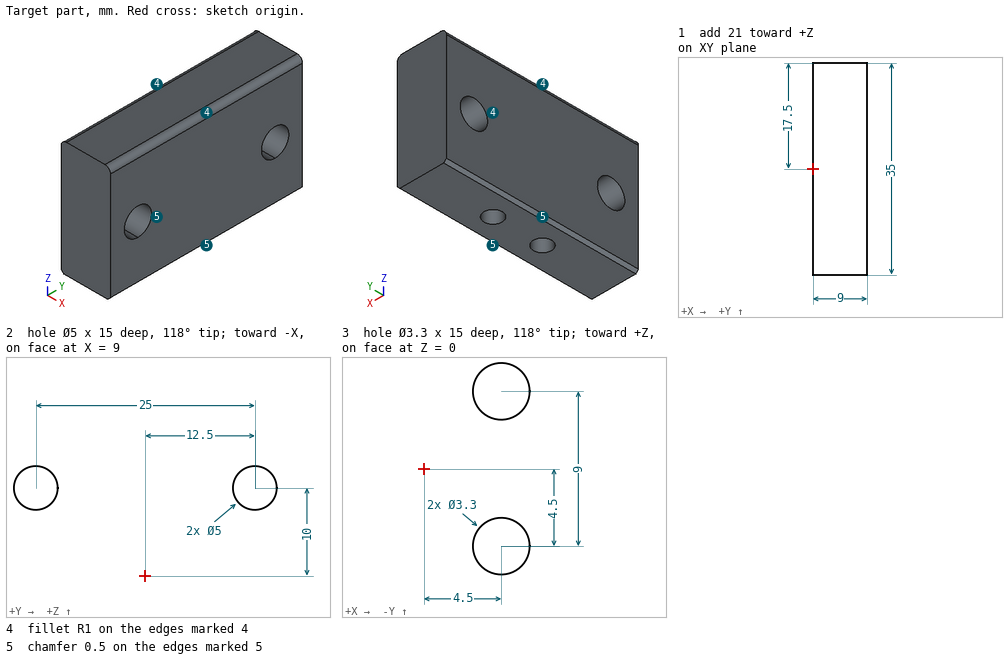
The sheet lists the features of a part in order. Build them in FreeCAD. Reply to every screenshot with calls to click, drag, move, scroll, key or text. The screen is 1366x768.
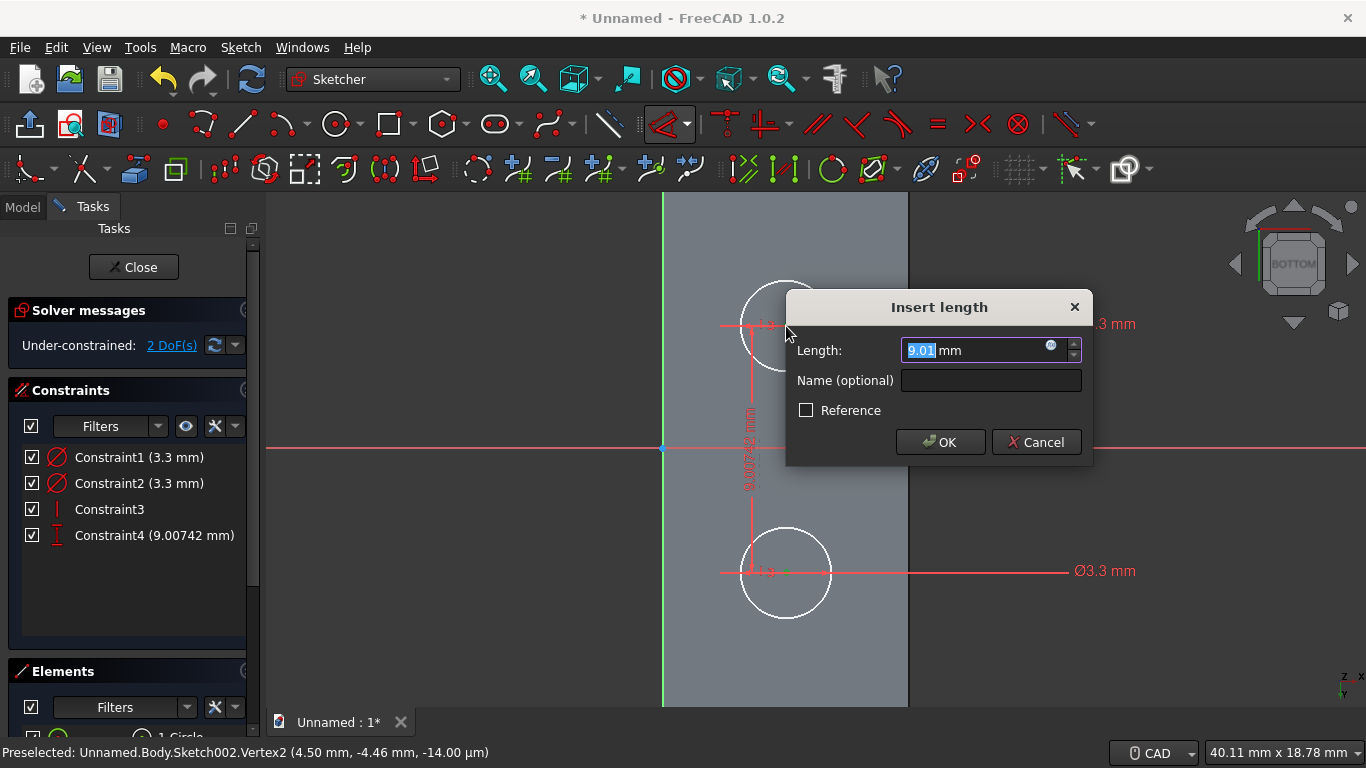
text(9)
key(Return)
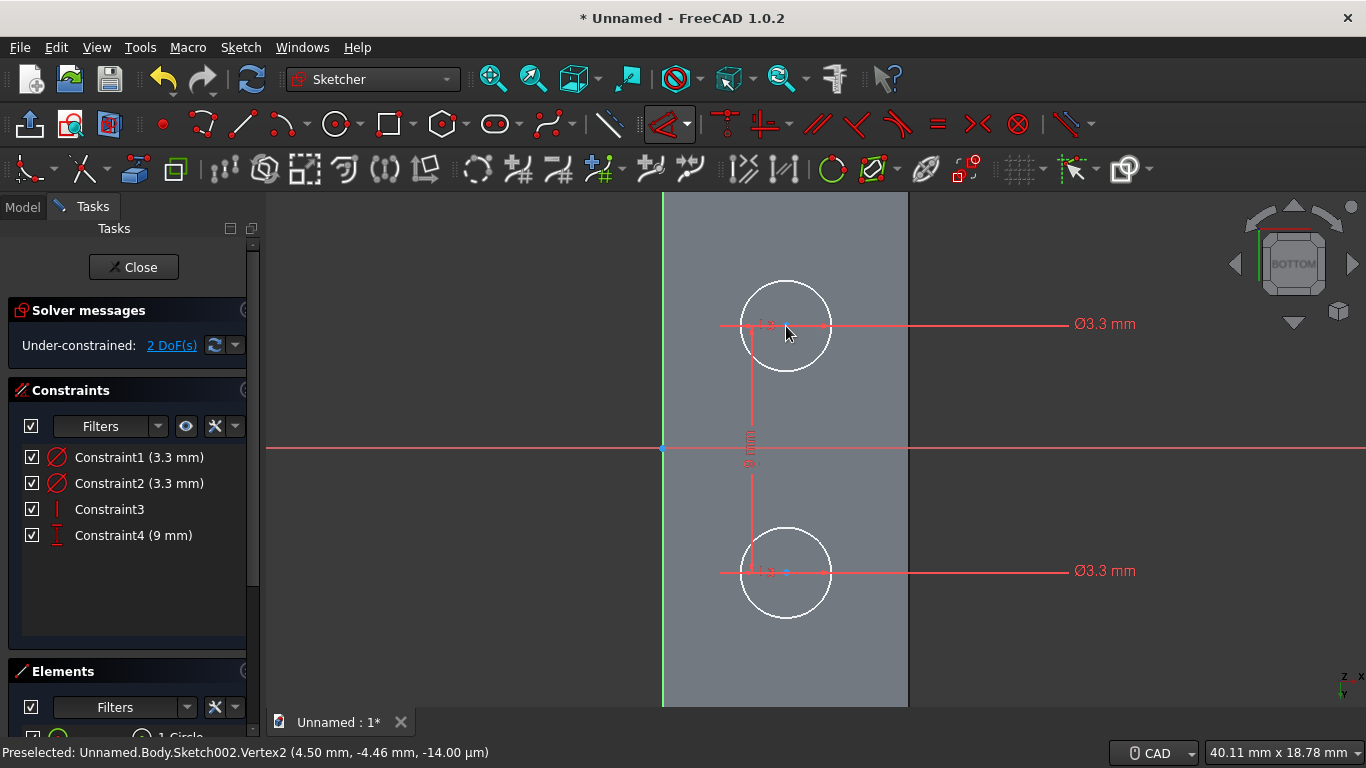
click(786, 573)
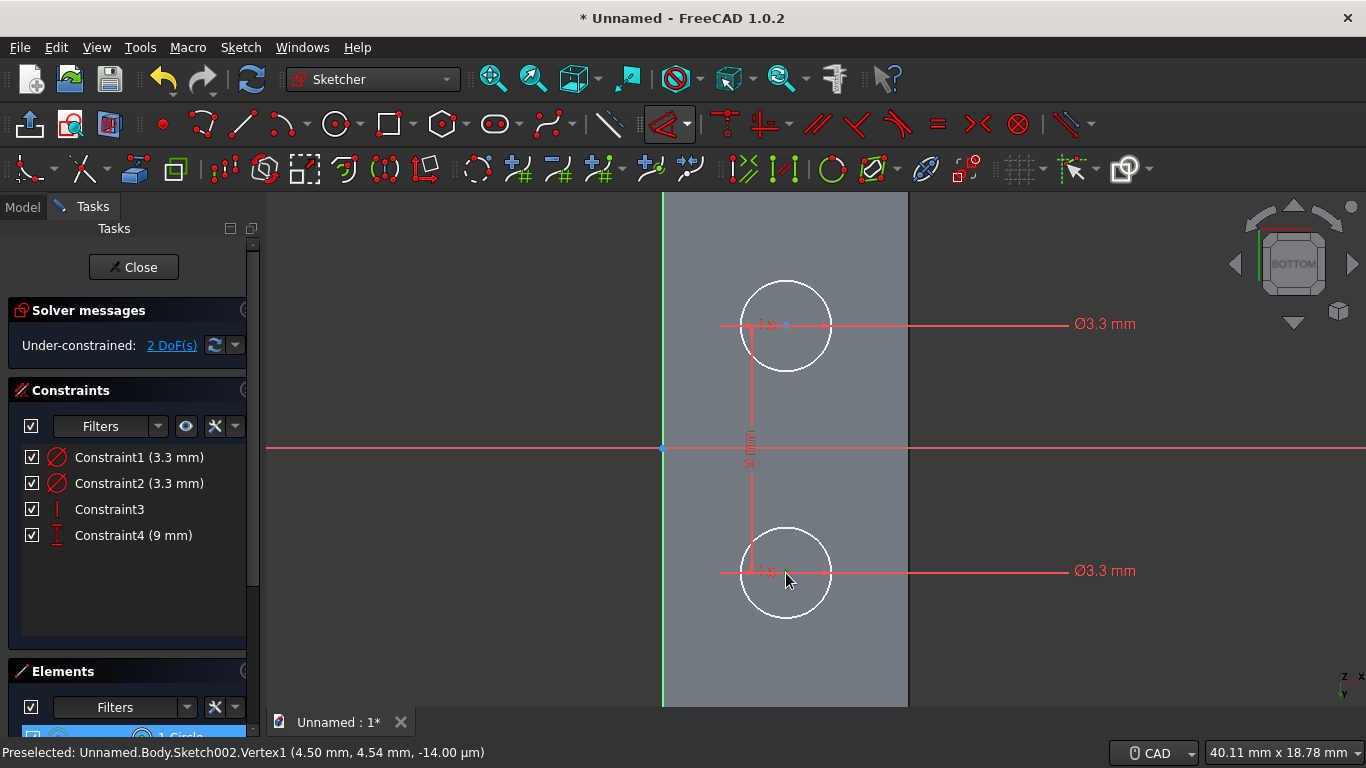
key(l)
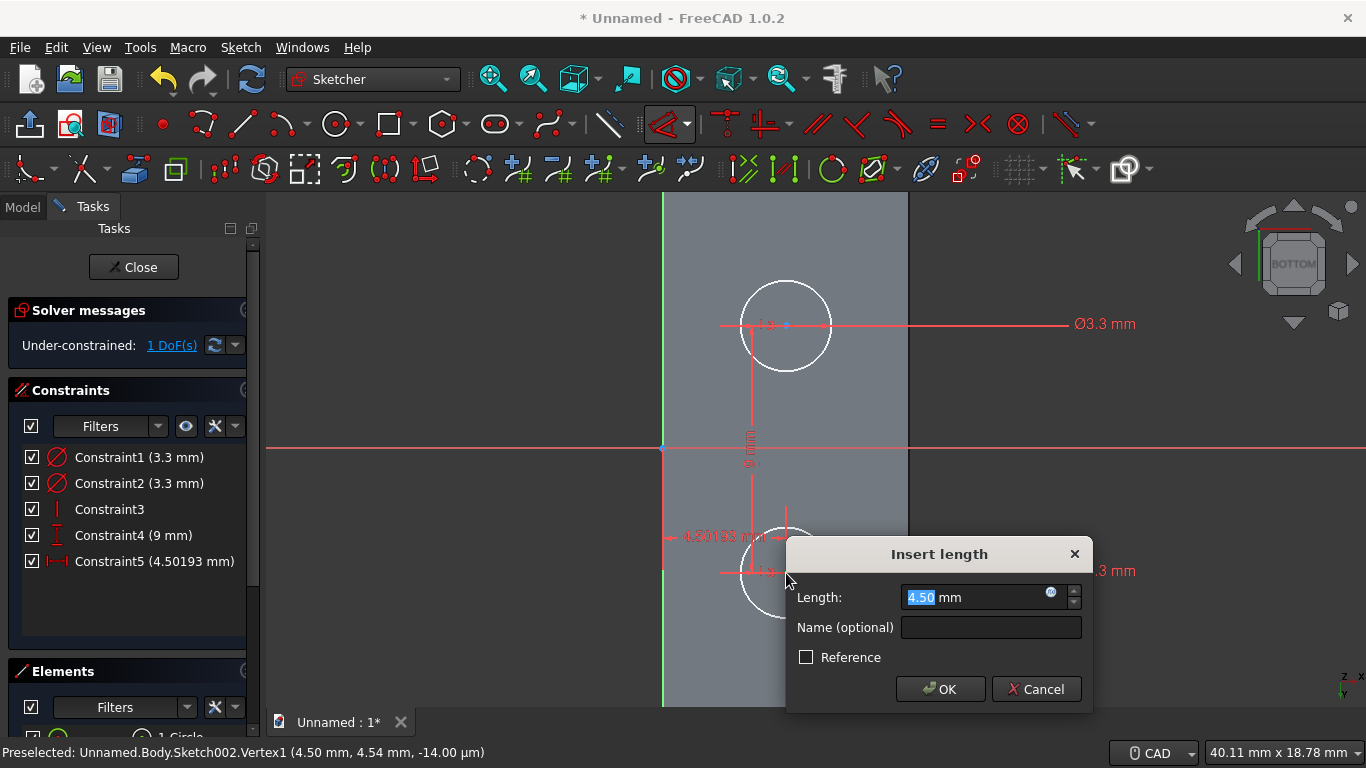
text(4.5)
key(Return)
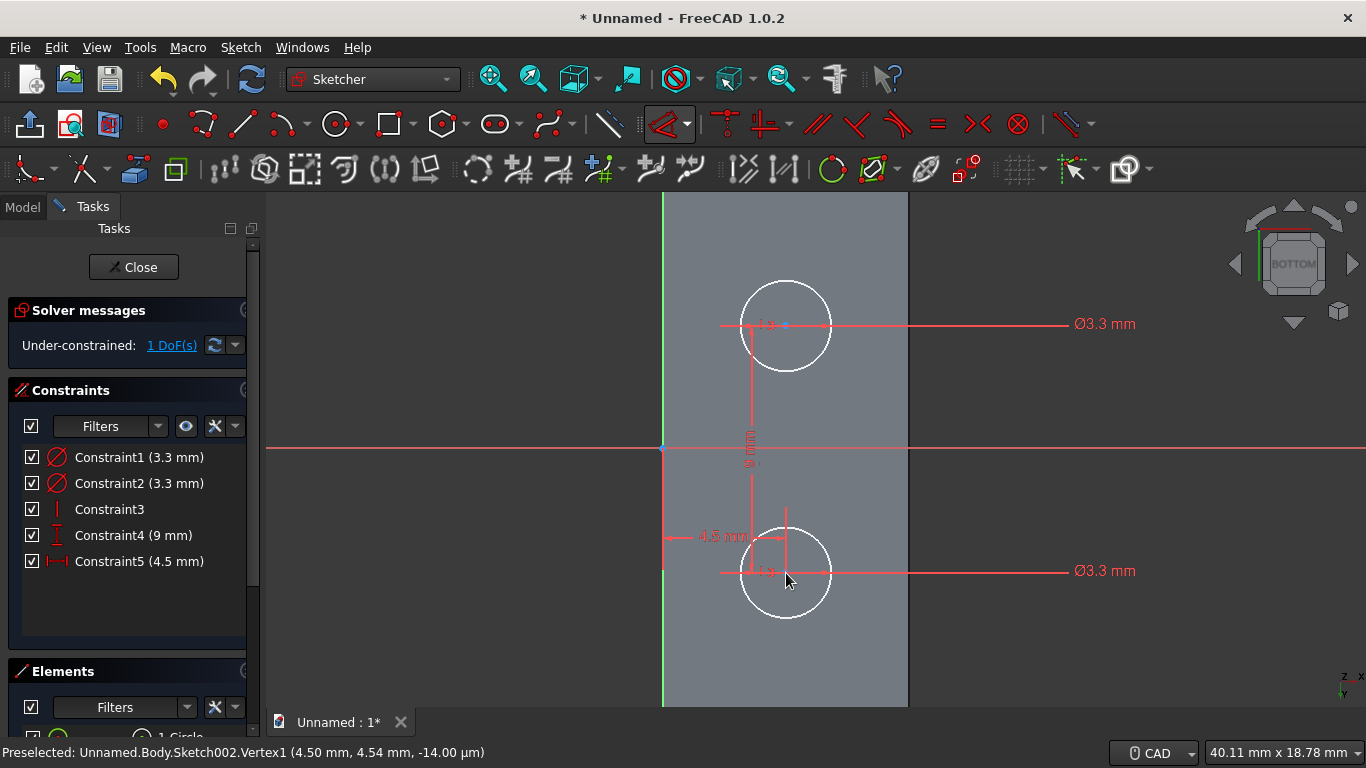
click(786, 573)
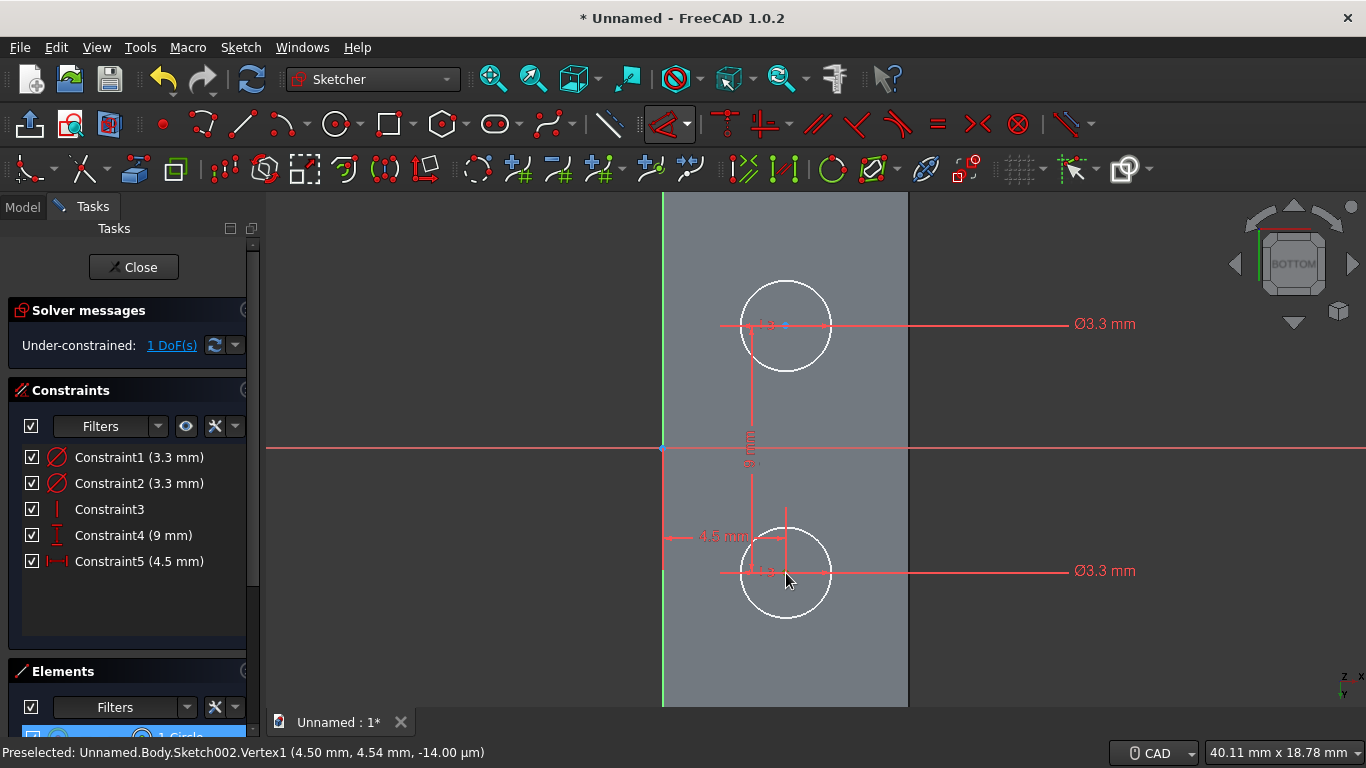
key(i)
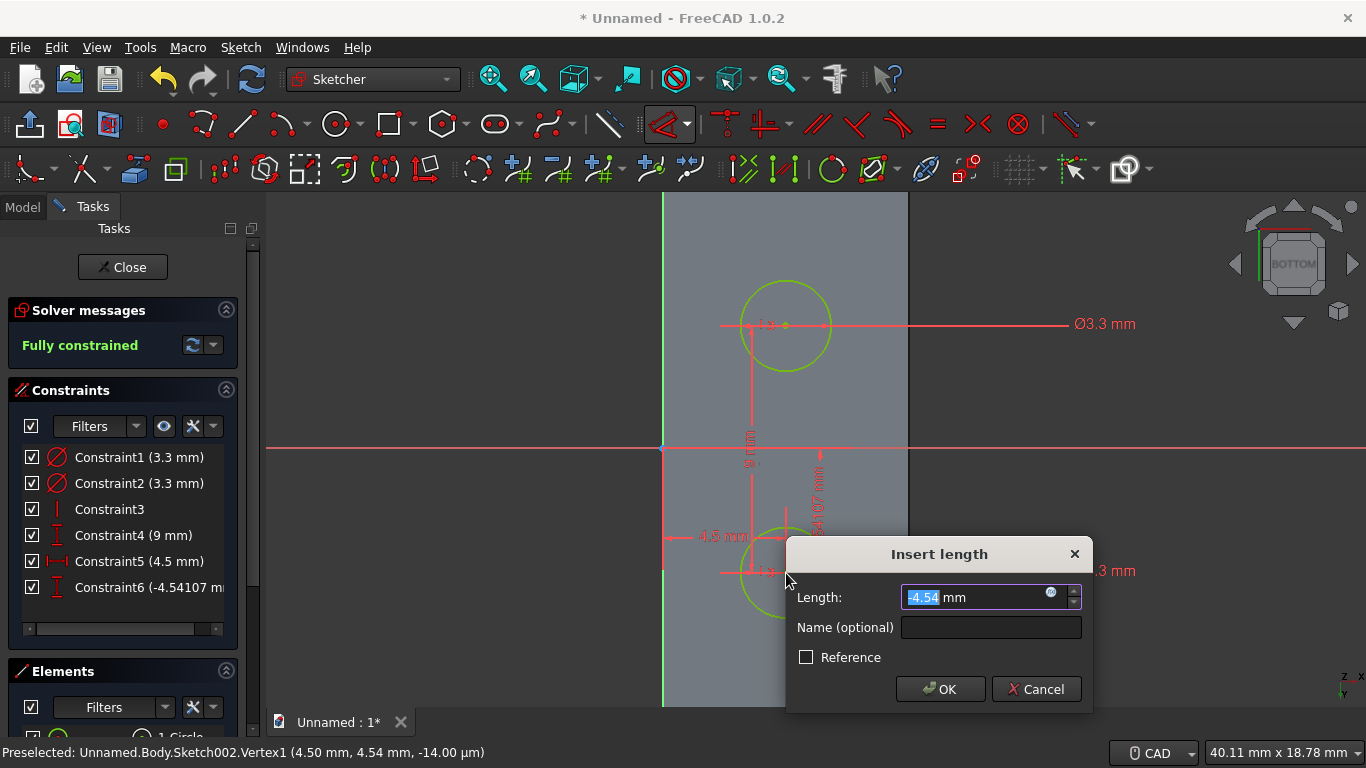
text(-4.5)
key(Return)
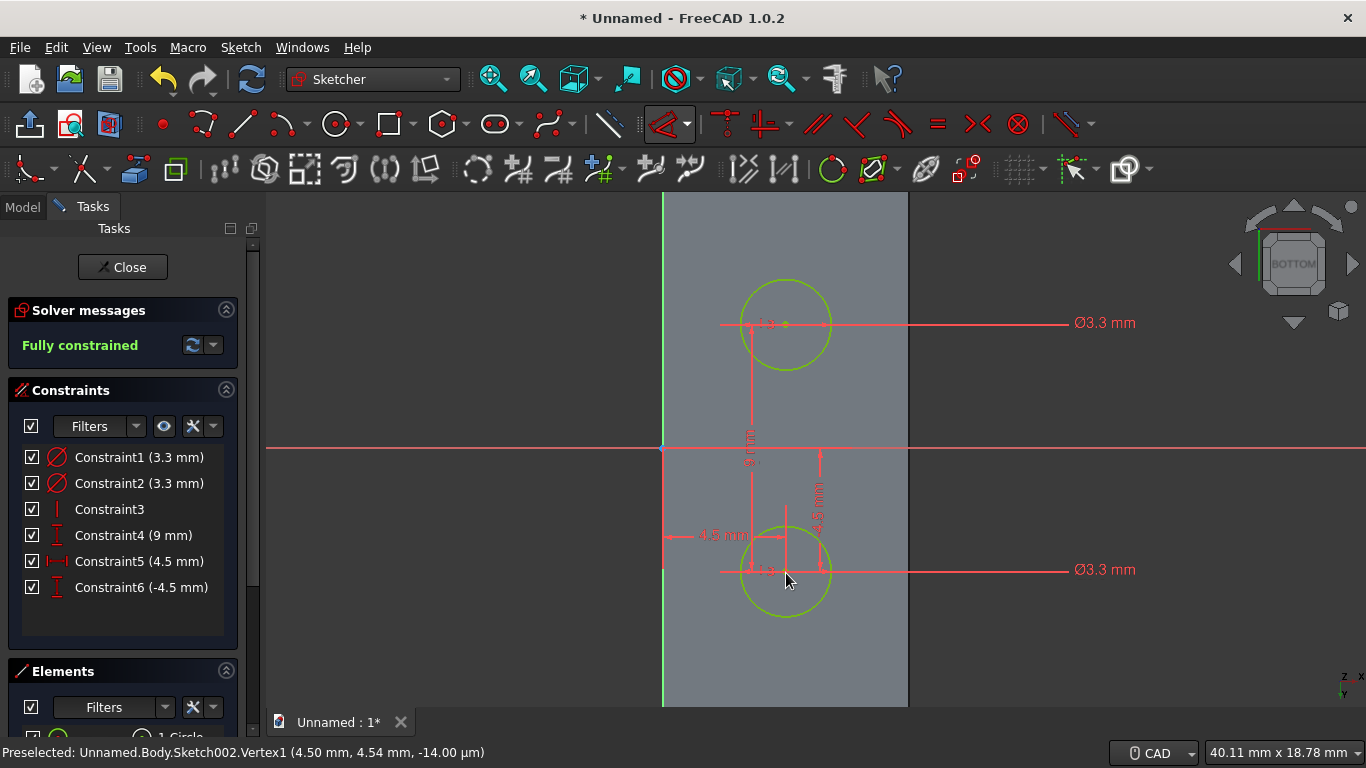
click(123, 267)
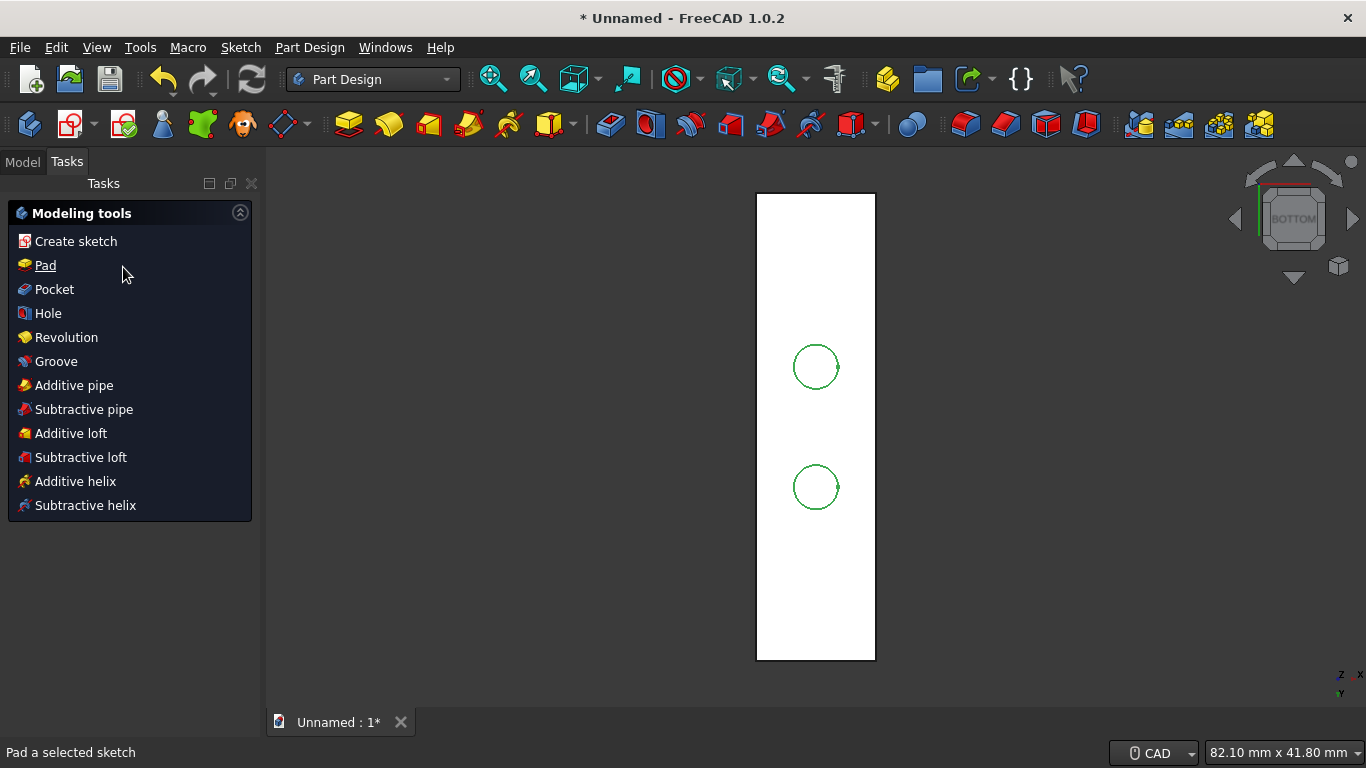
click(652, 124)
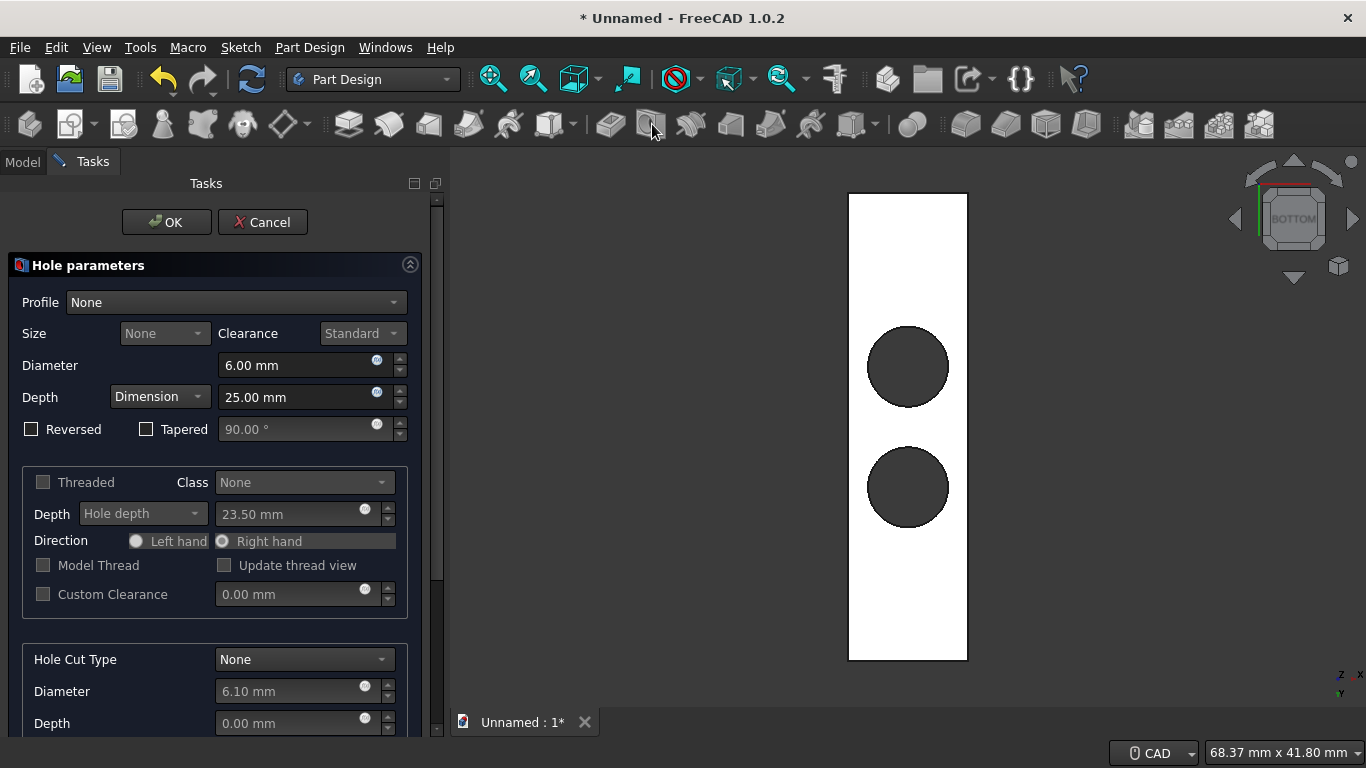
triple_click(305, 365)